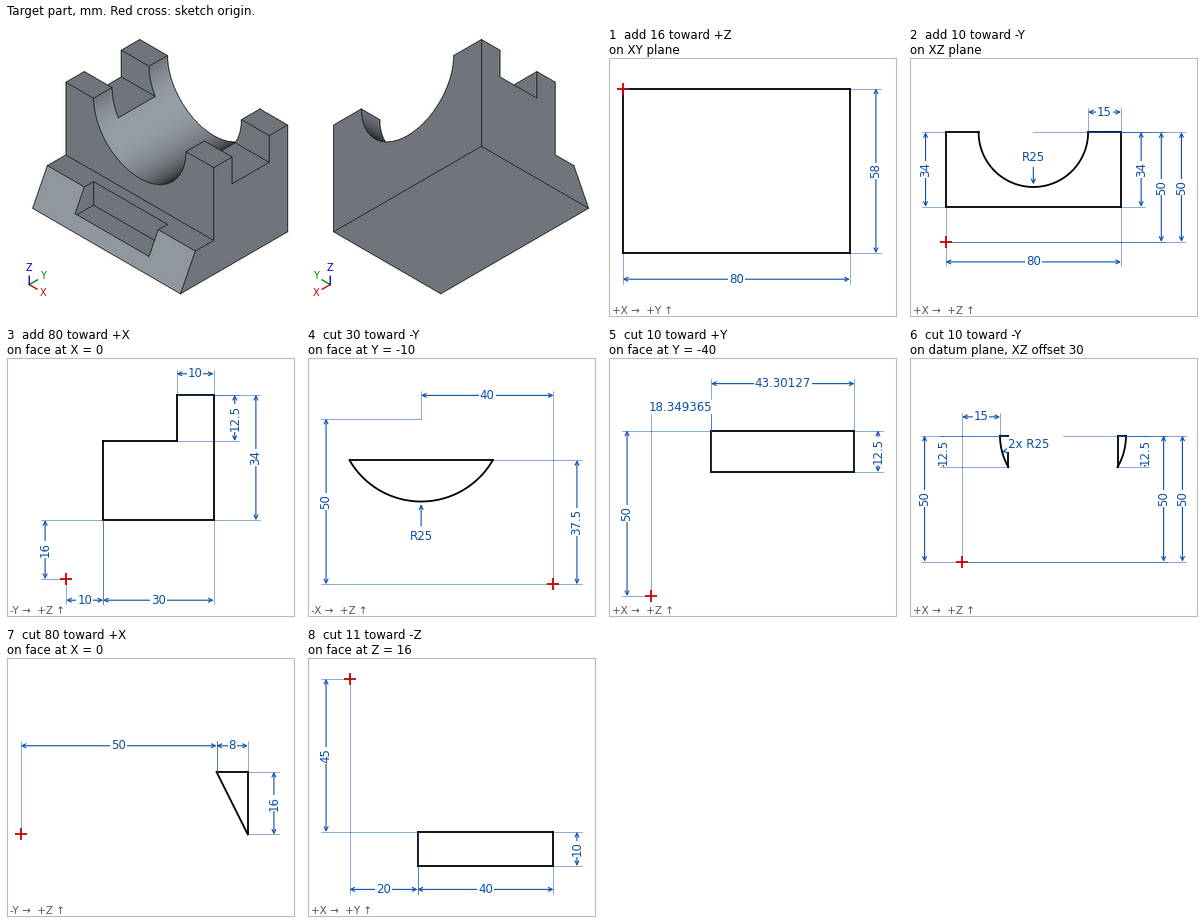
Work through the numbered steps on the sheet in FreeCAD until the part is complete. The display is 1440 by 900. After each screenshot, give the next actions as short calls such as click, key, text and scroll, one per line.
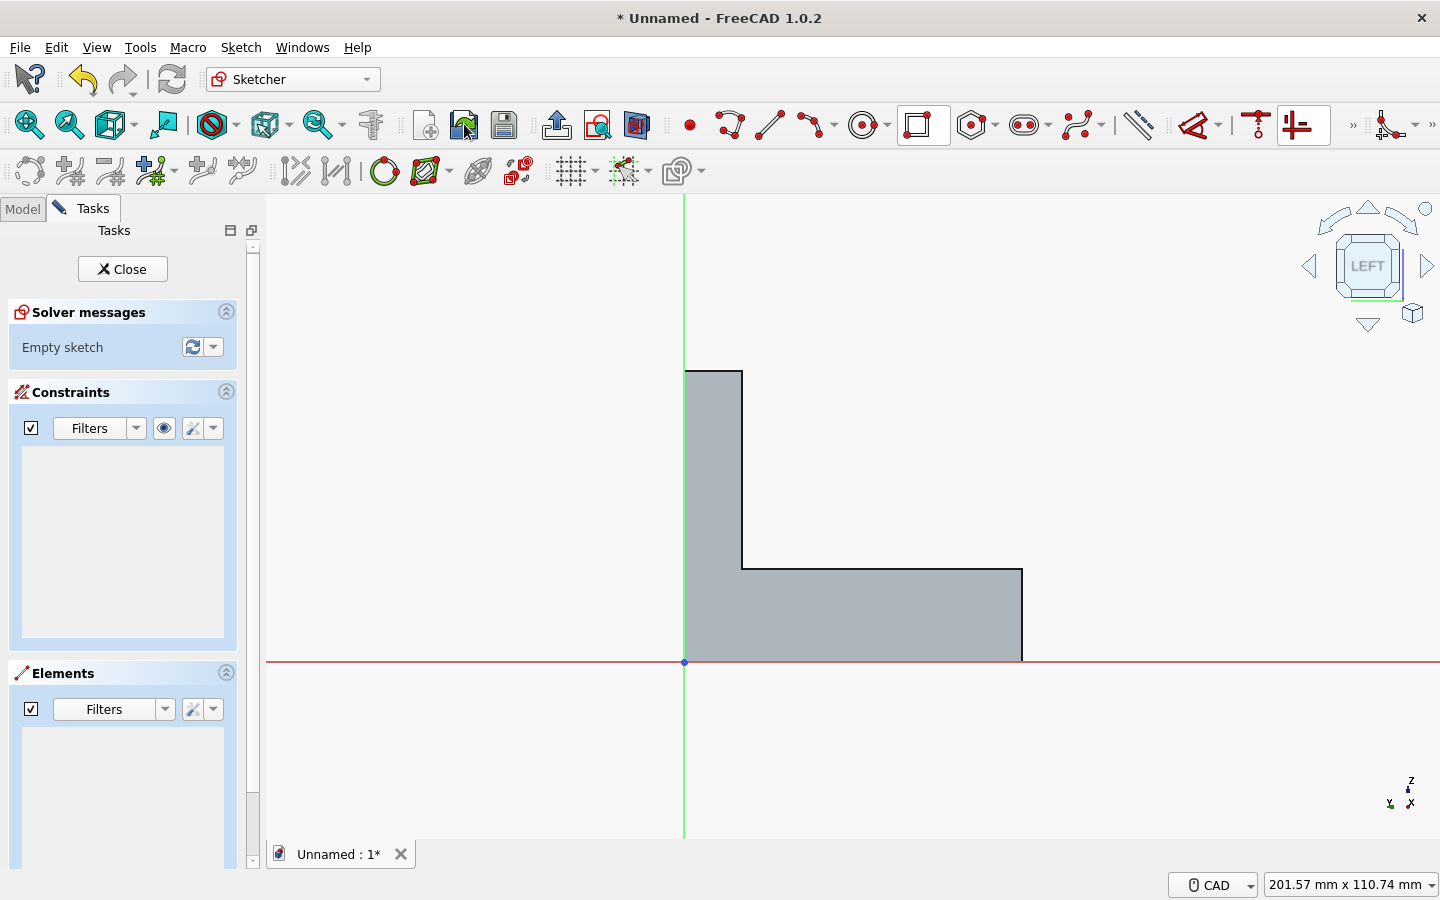
scroll(833, 517, up, 2)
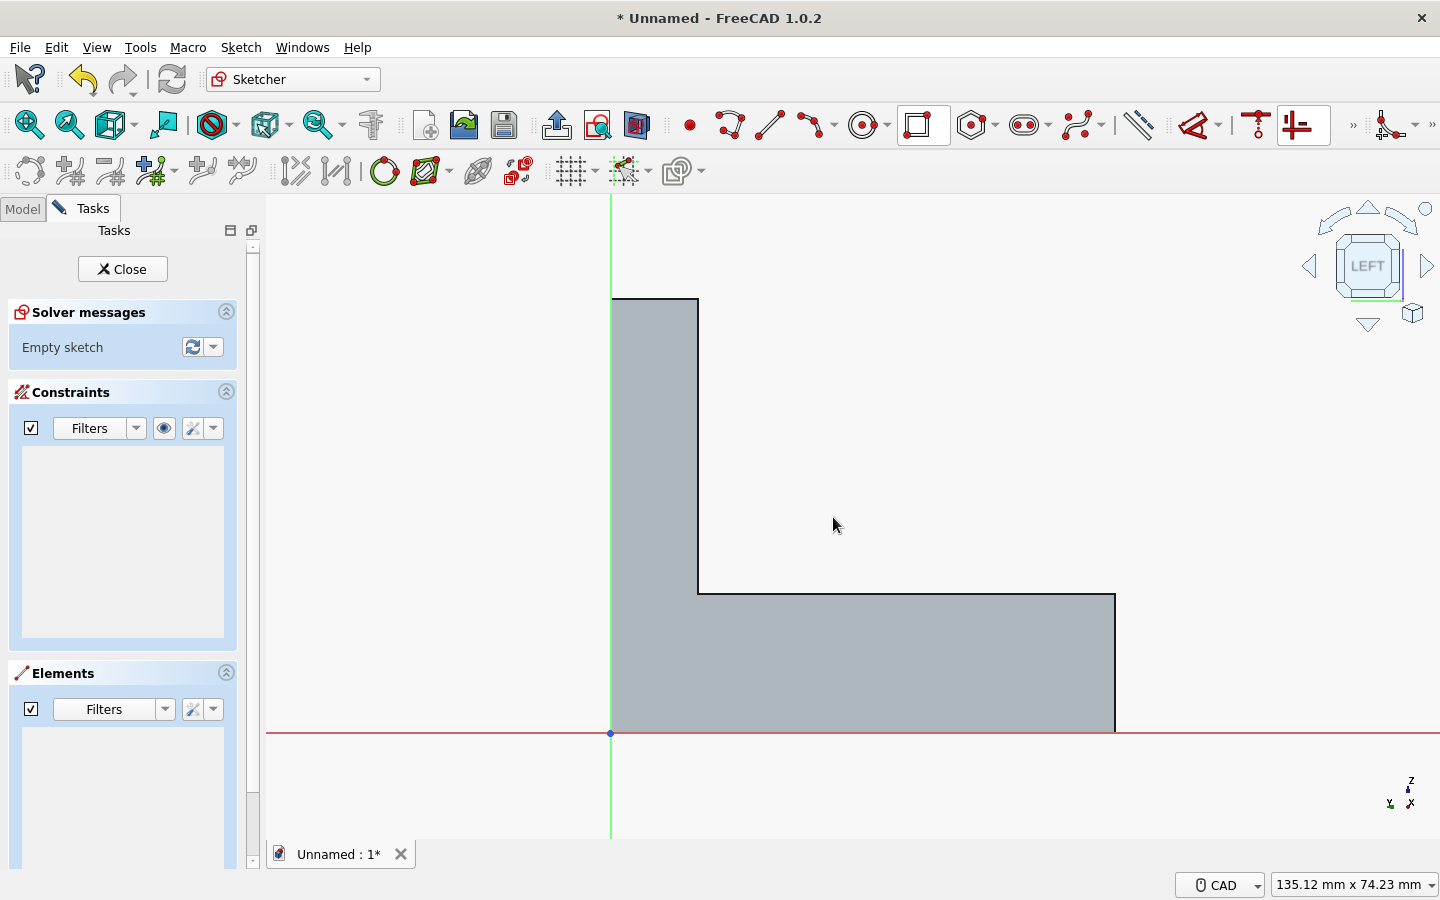
click(730, 126)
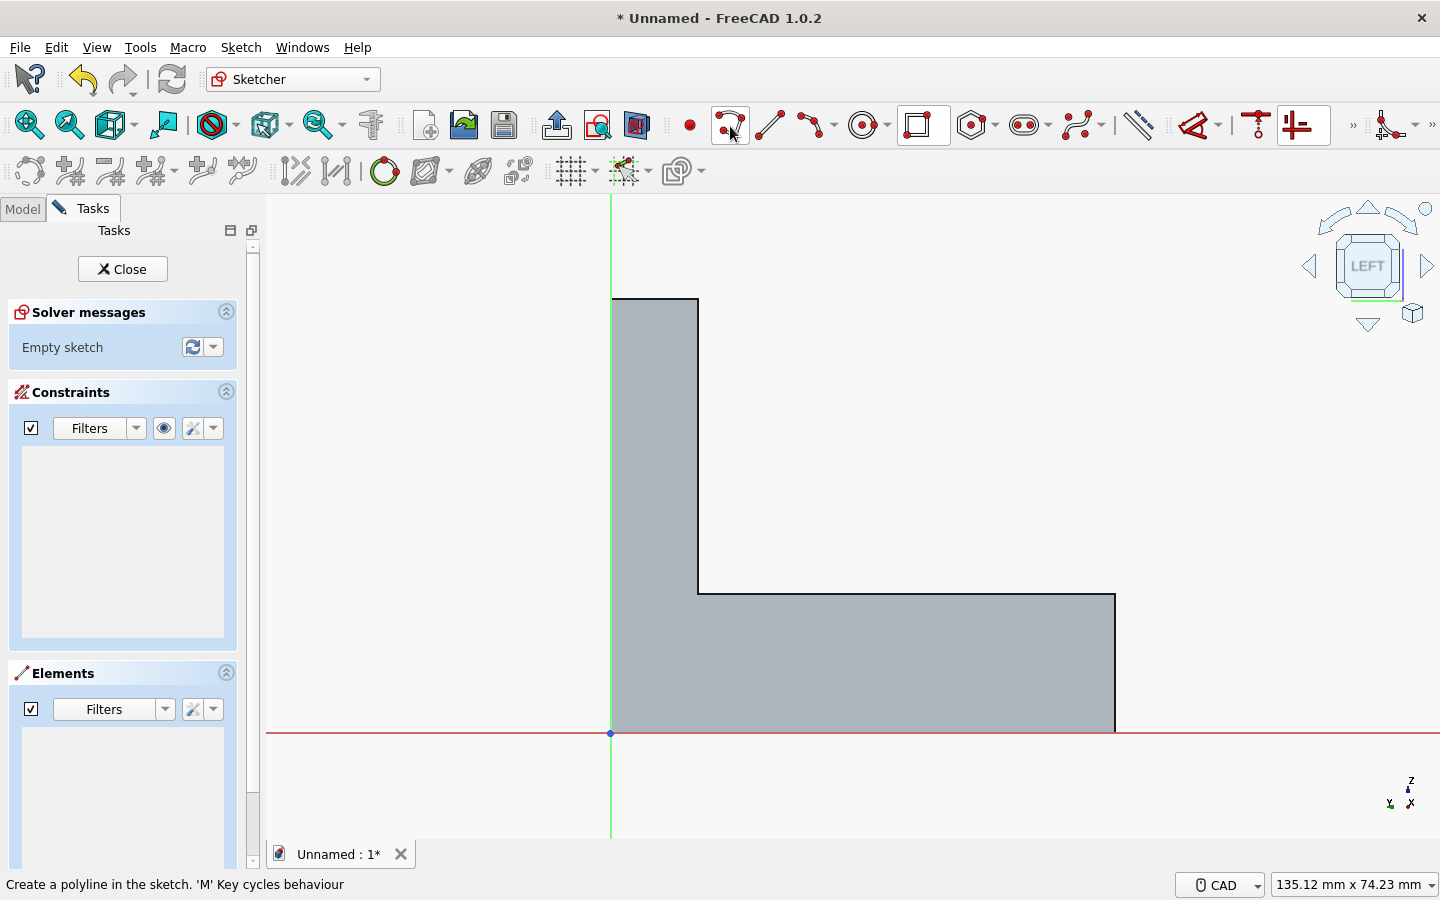
click(698, 594)
click(958, 594)
click(958, 299)
click(871, 299)
click(871, 407)
click(698, 407)
click(698, 595)
key(Escape)
key(Escape)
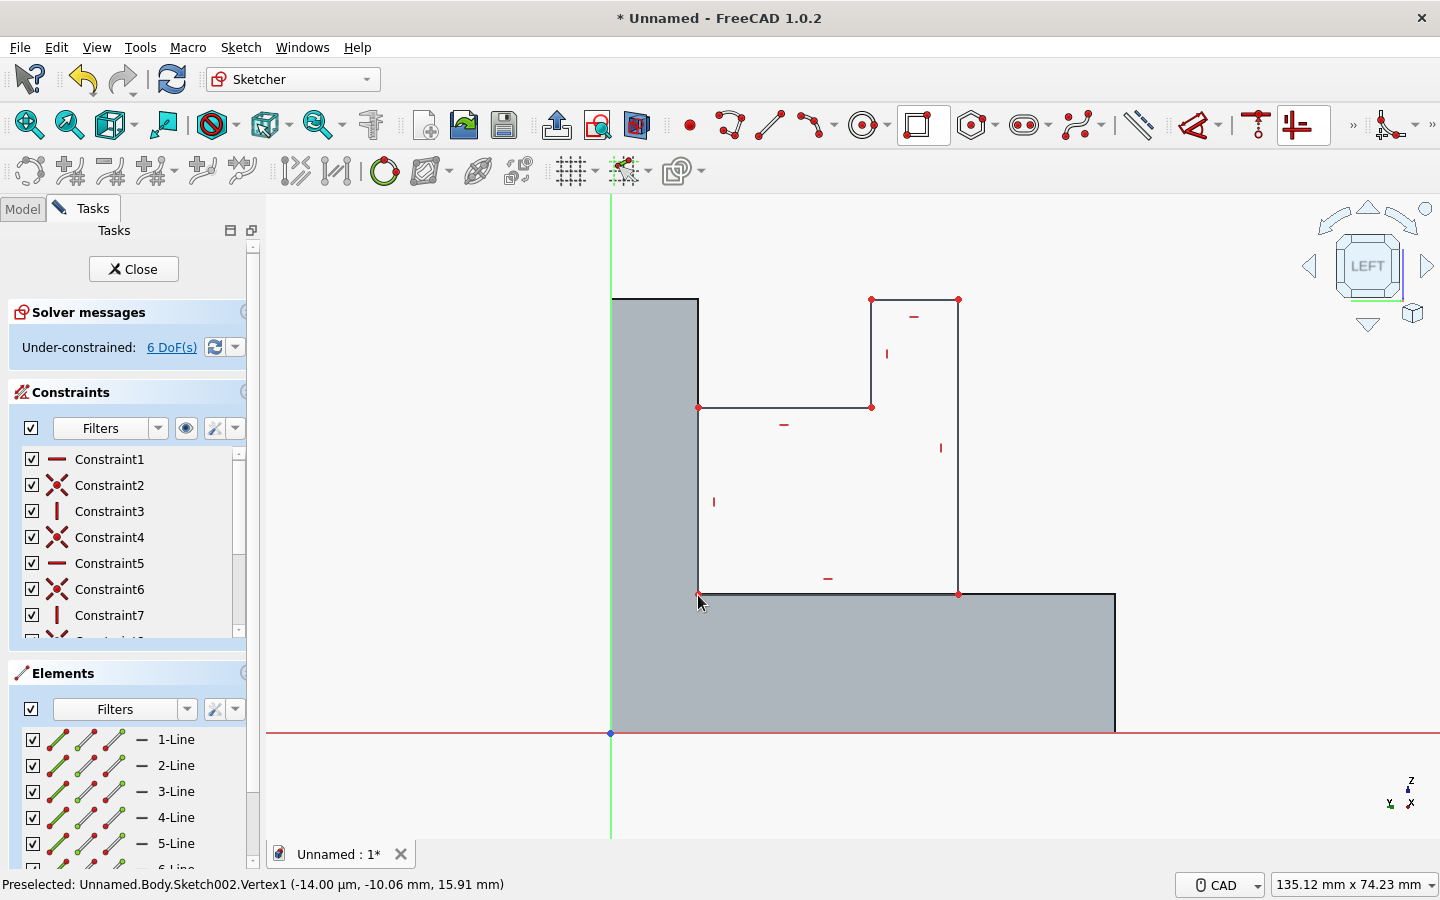
click(1194, 126)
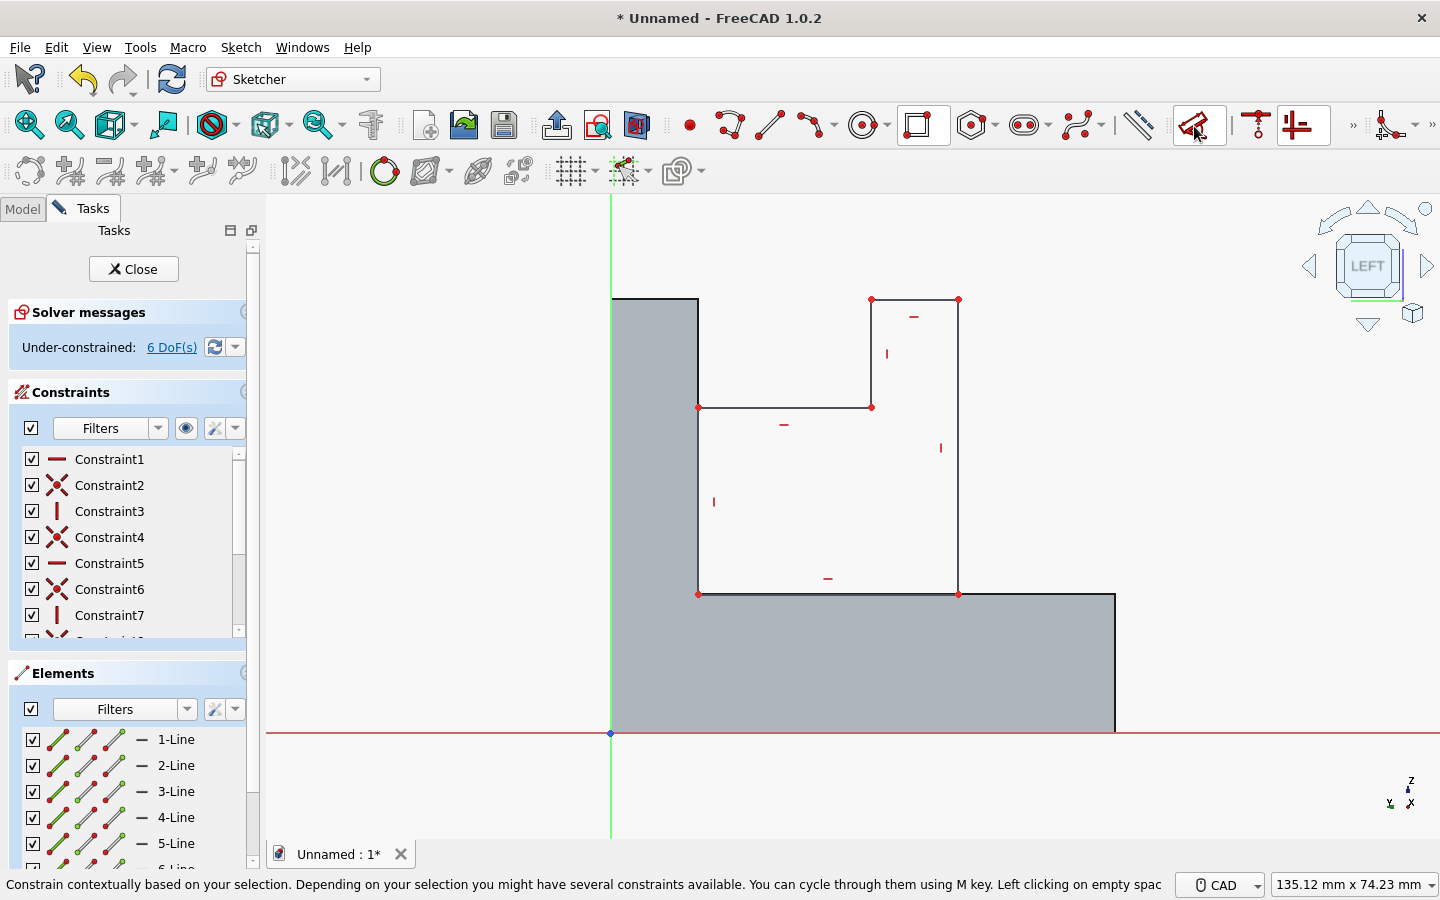
click(776, 595)
click(828, 629)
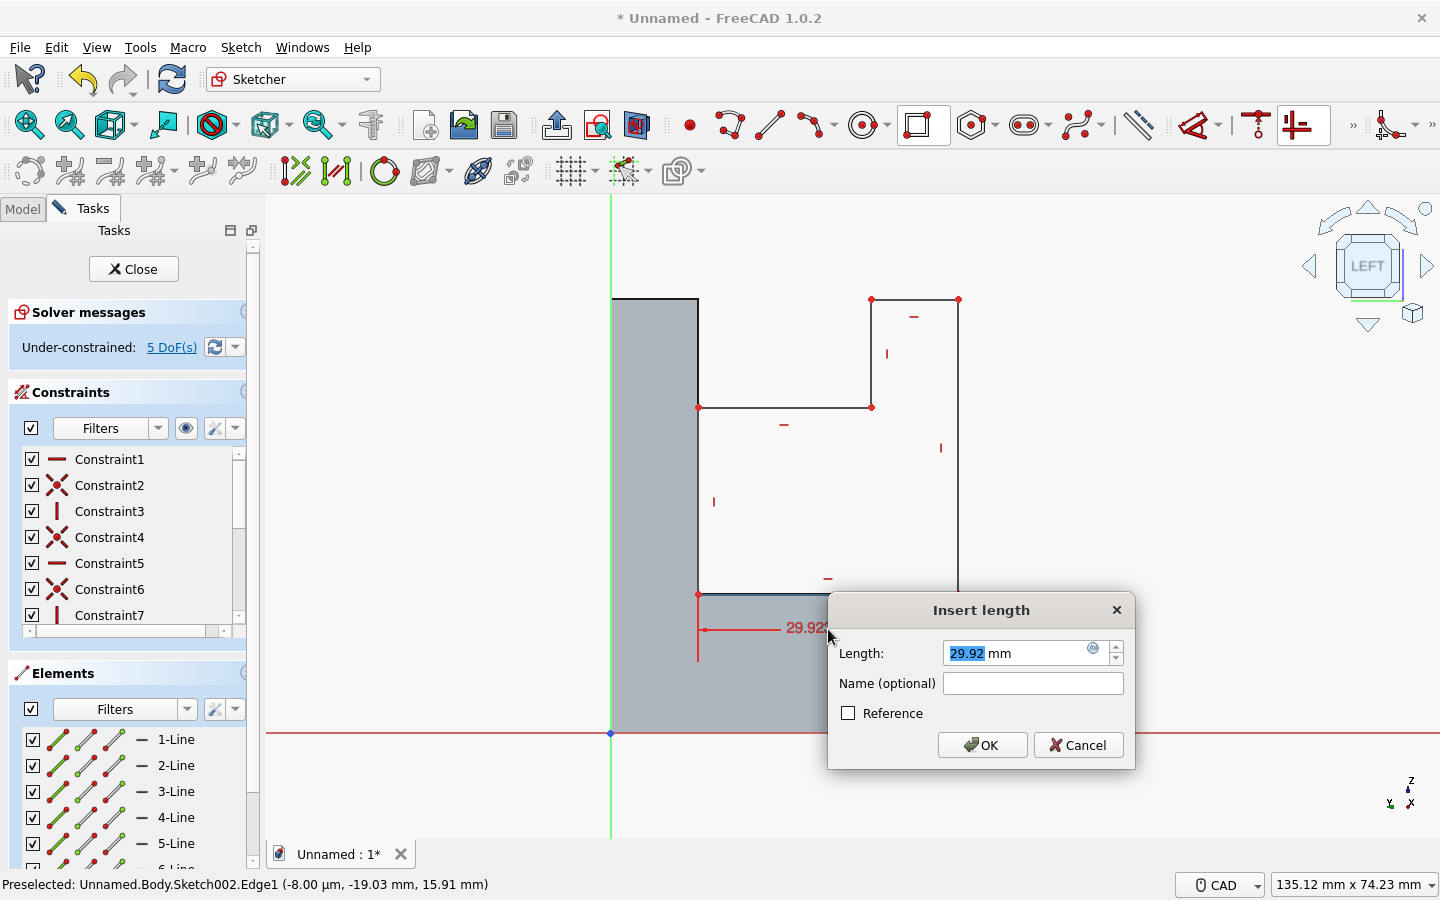
text(30)
key(Return)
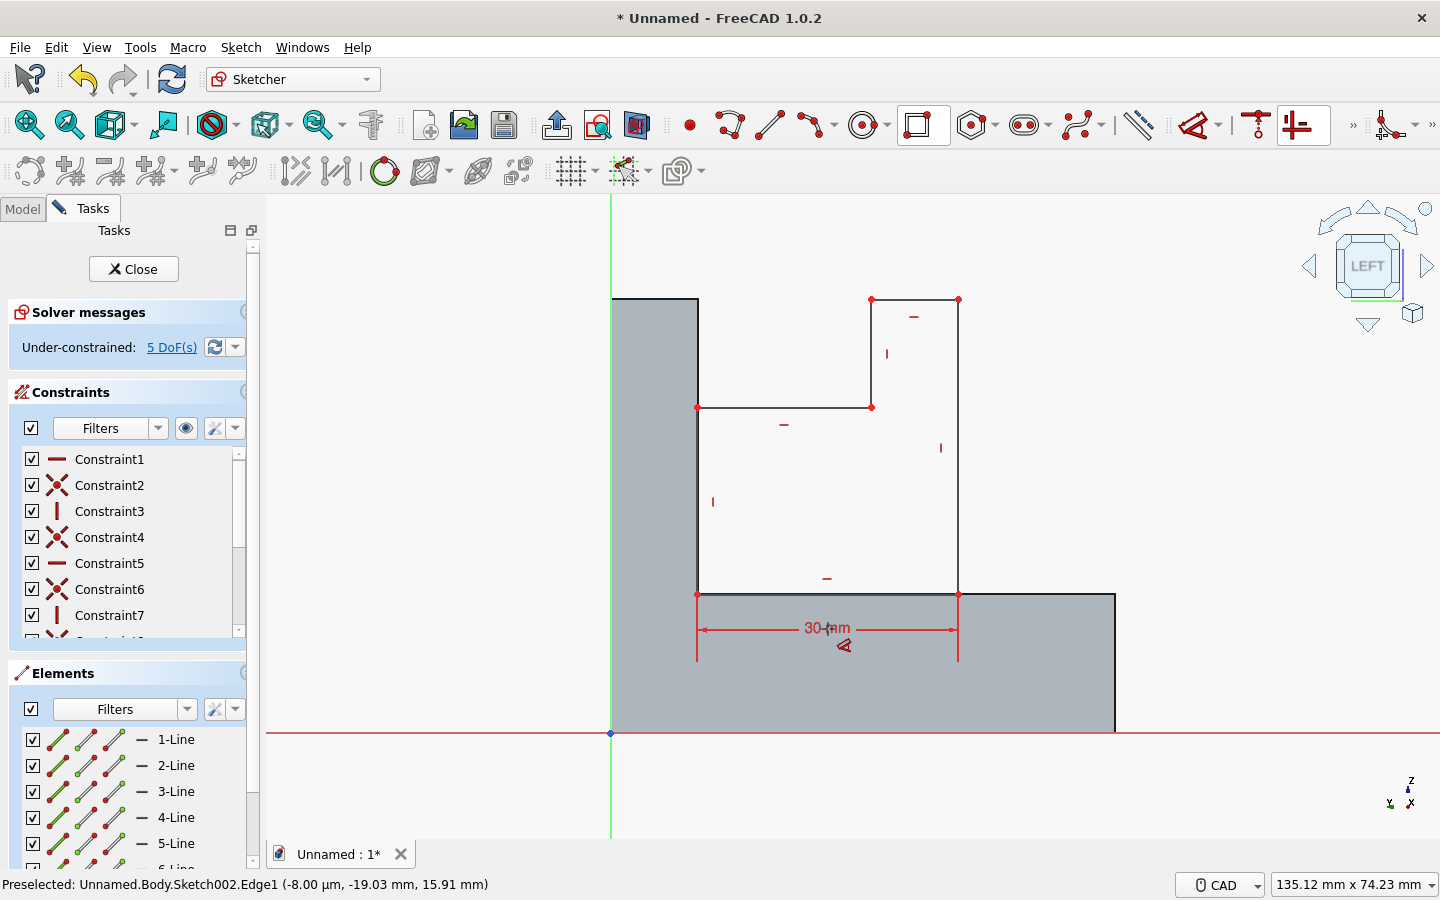
click(958, 506)
click(992, 447)